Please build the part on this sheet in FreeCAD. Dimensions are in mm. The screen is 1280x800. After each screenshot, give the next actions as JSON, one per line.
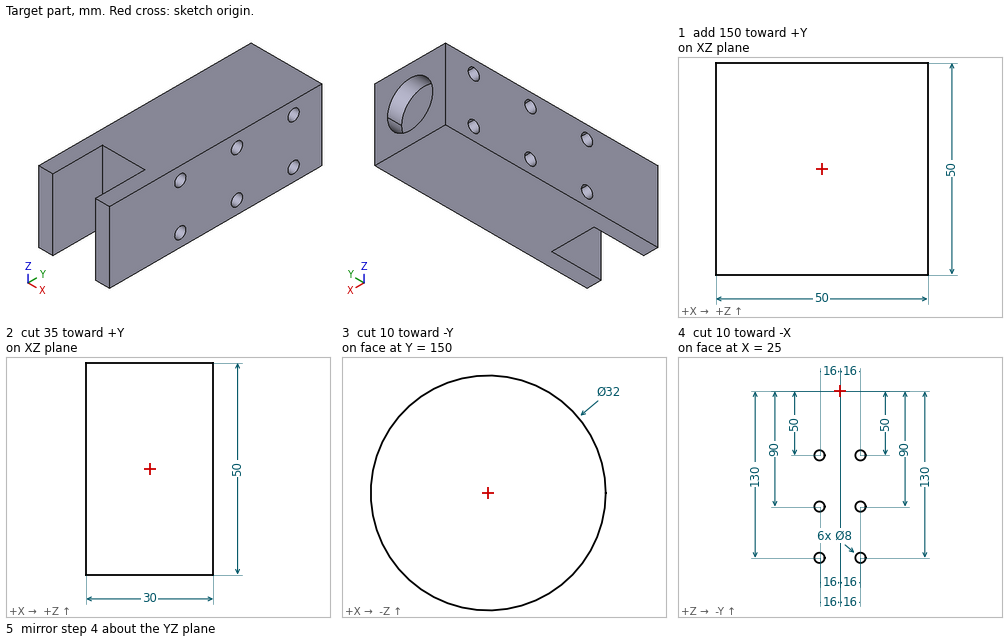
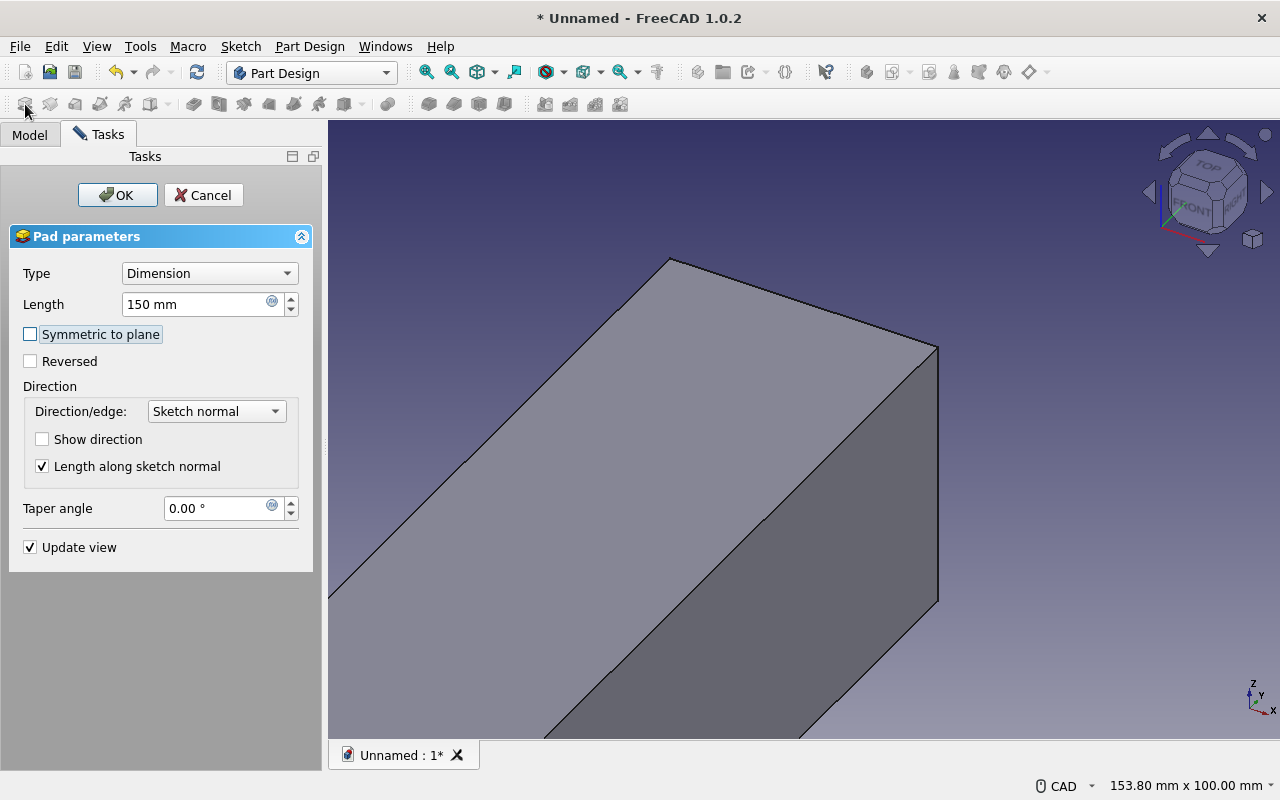
{"action": "left_click", "coordinate": [31, 361]}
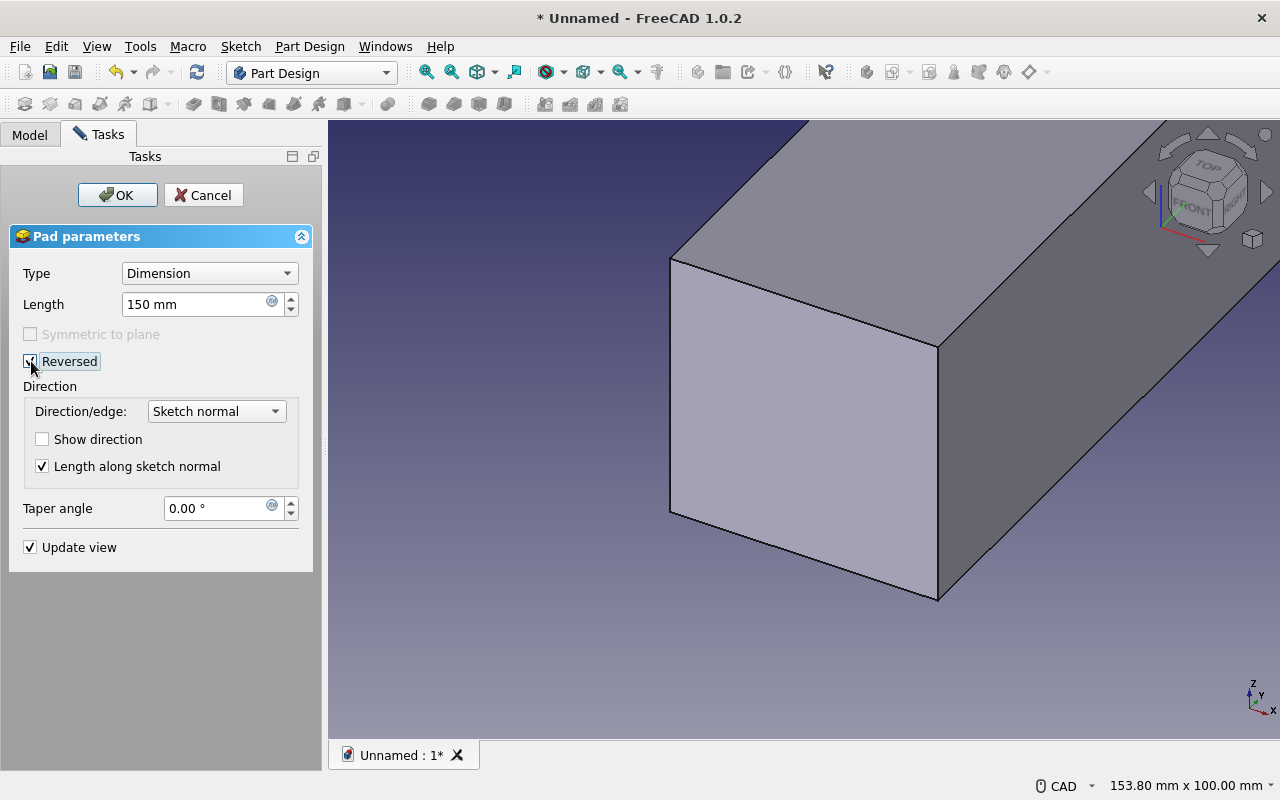
{"action": "left_click", "coordinate": [118, 195]}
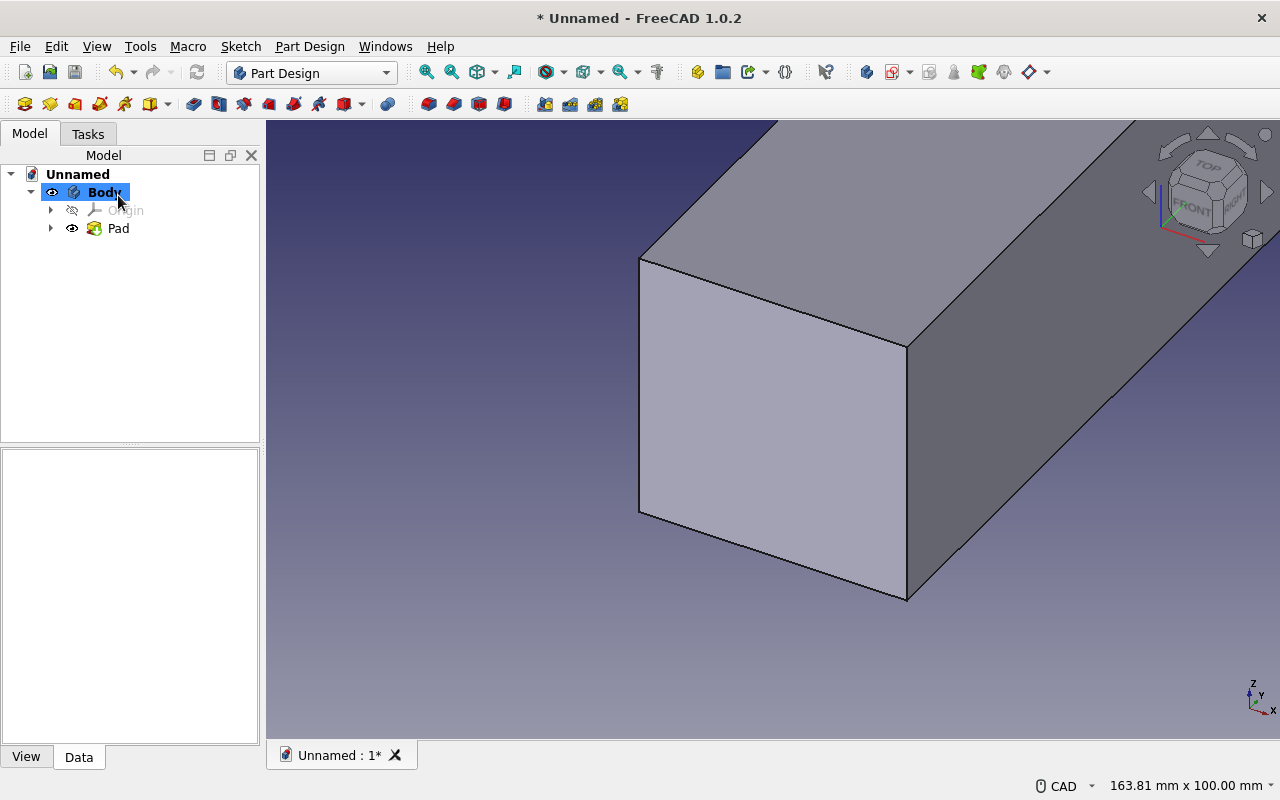
{"action": "left_click", "coordinate": [427, 72]}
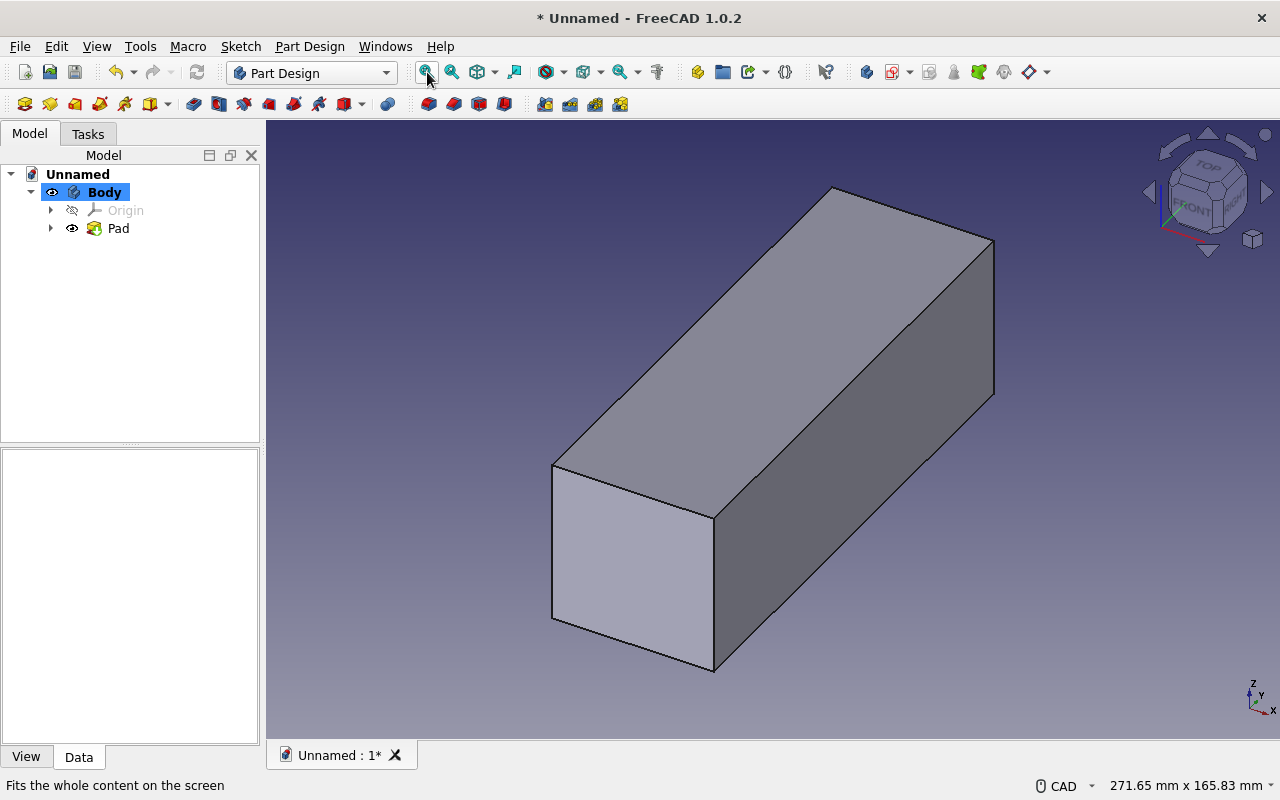
{"action": "left_click", "coordinate": [892, 72]}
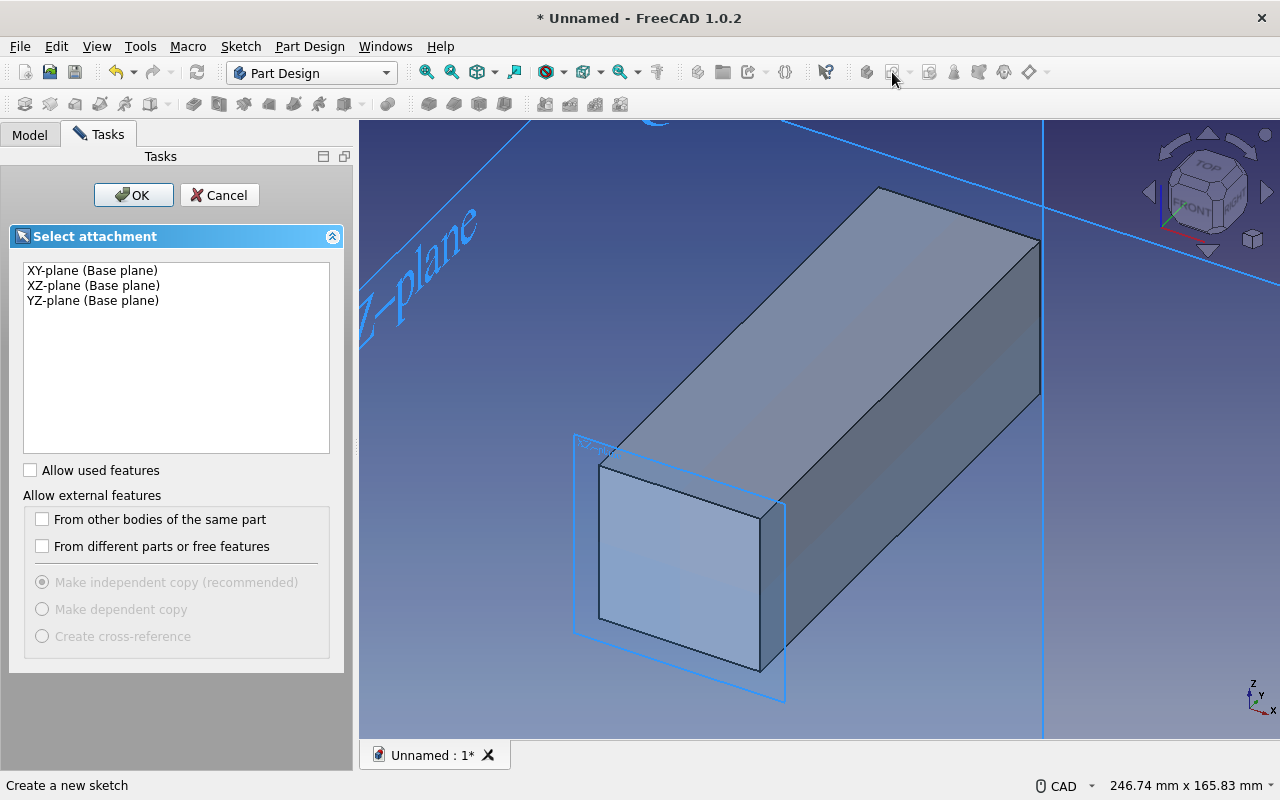
{"action": "left_click", "coordinate": [84, 286]}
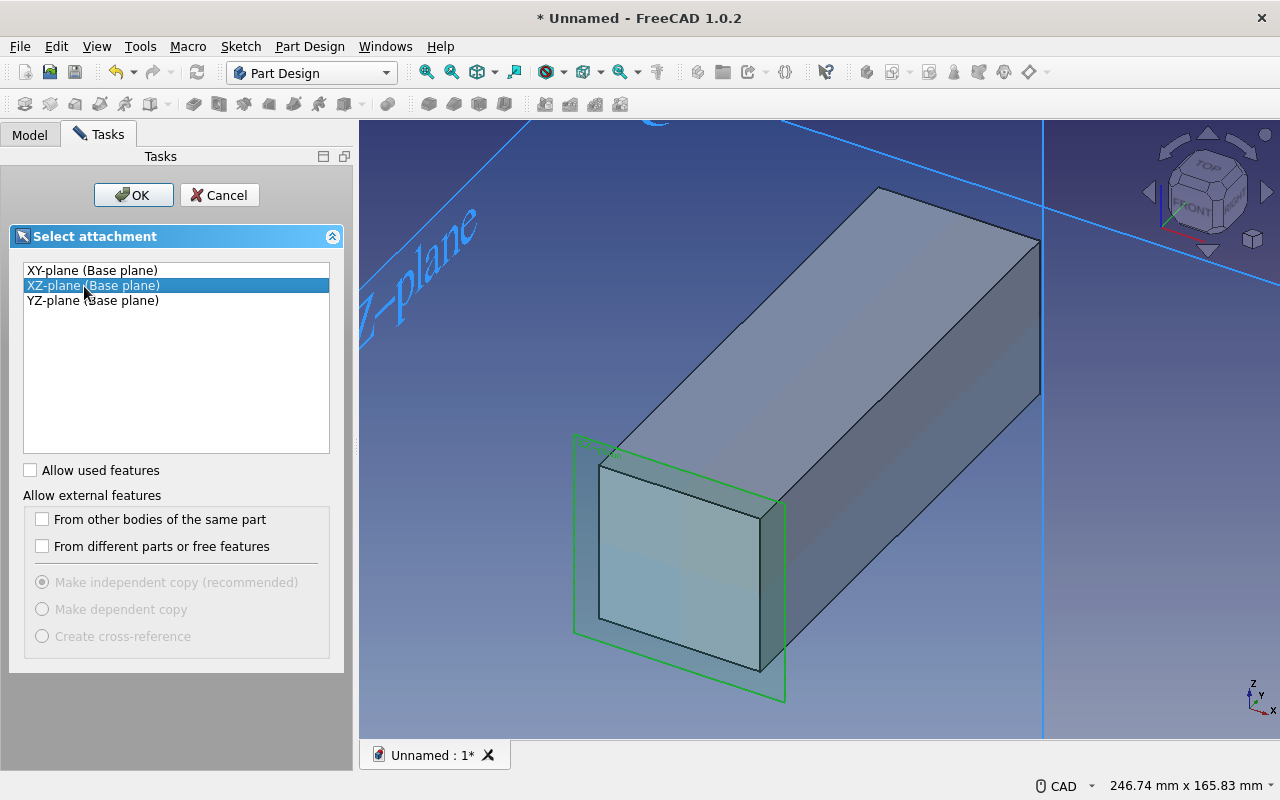
{"action": "left_click", "coordinate": [134, 195]}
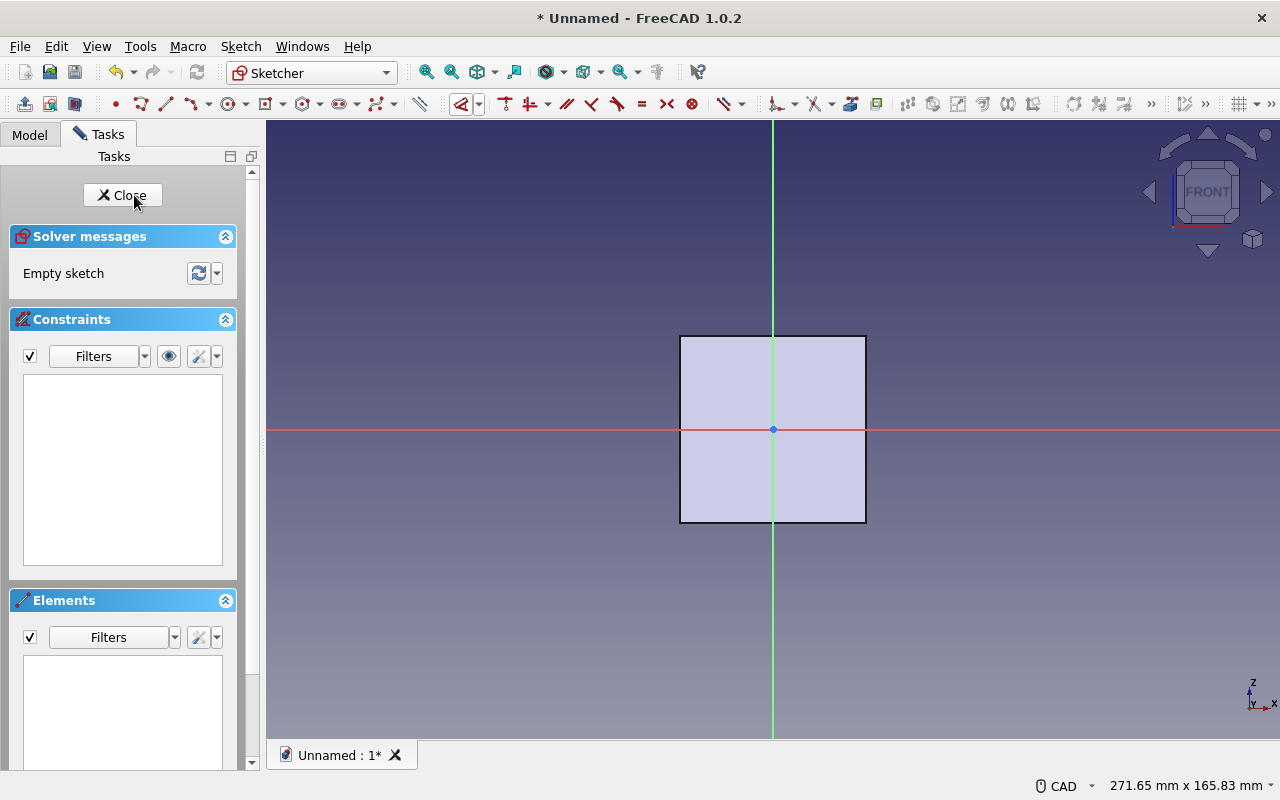
{"action": "scroll", "coordinate": [829, 430], "scroll_direction": "up", "scroll_amount": 4}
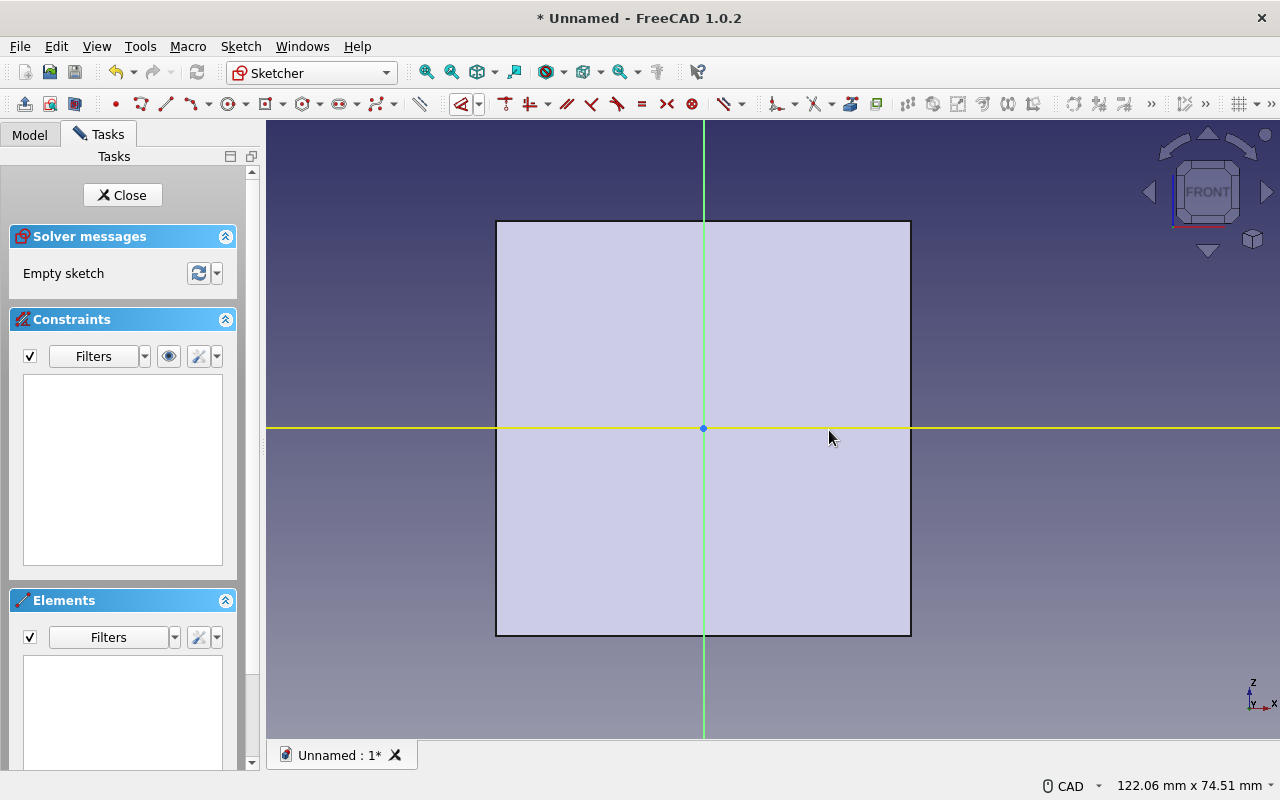
{"action": "left_click", "coordinate": [264, 104]}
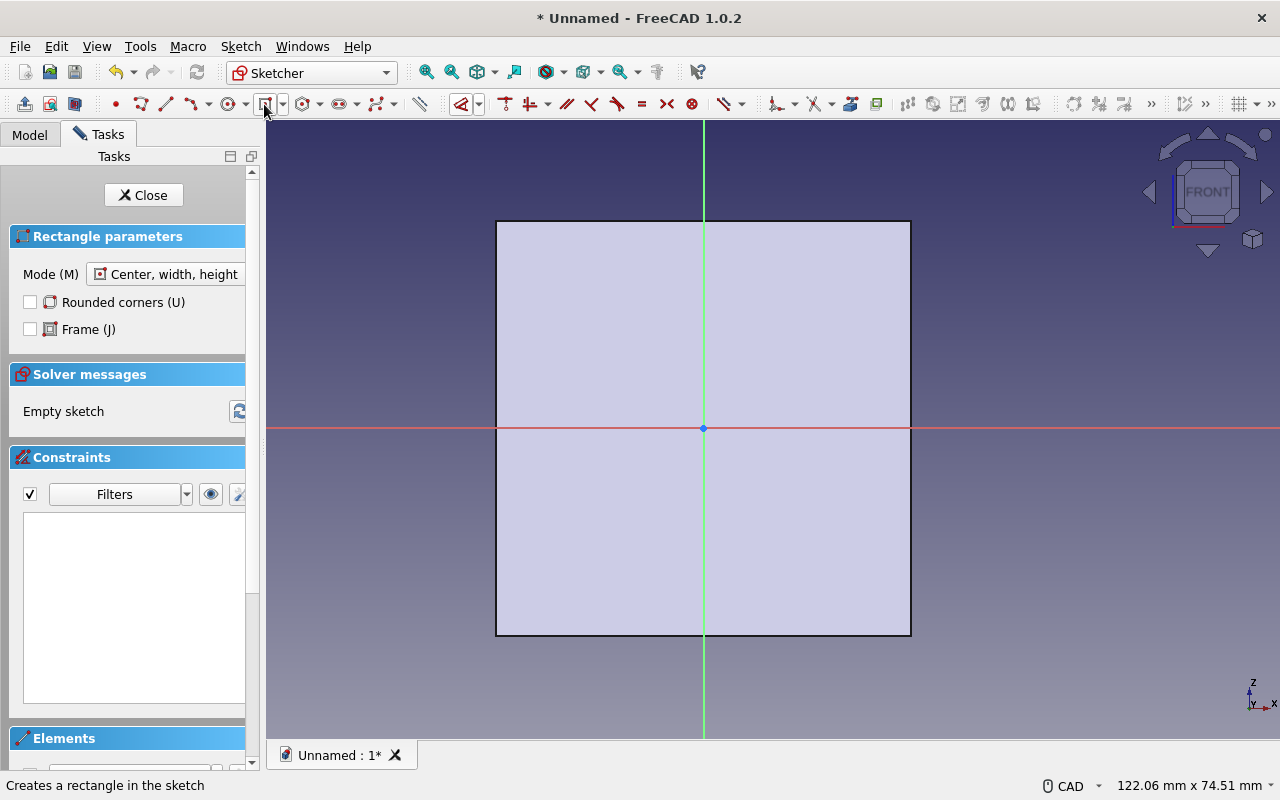
{"action": "left_click", "coordinate": [704, 428]}
{"action": "mouse_move", "coordinate": [828, 221]}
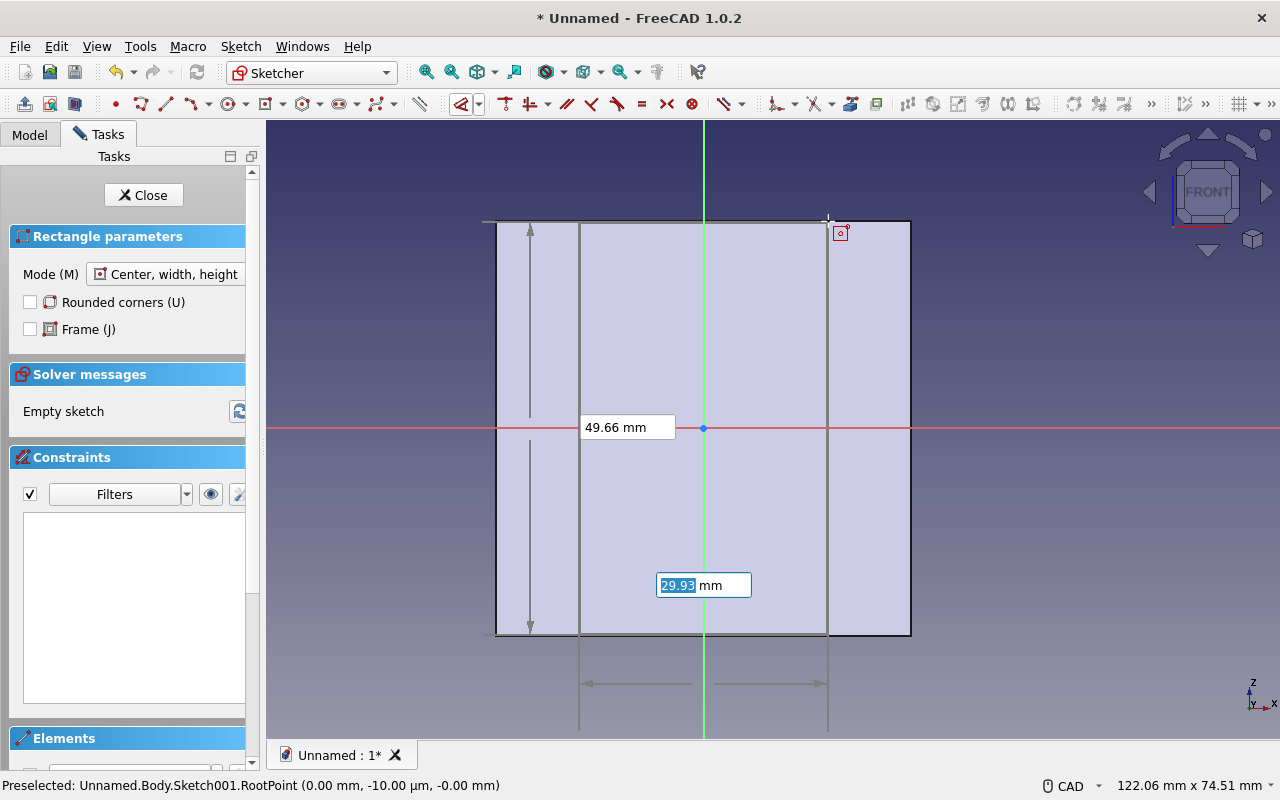
{"action": "type", "text": "30"}
{"action": "key", "text": "Tab"}
{"action": "type", "text": "50"}
{"action": "key", "text": "Return"}
{"action": "key", "text": "Escape"}